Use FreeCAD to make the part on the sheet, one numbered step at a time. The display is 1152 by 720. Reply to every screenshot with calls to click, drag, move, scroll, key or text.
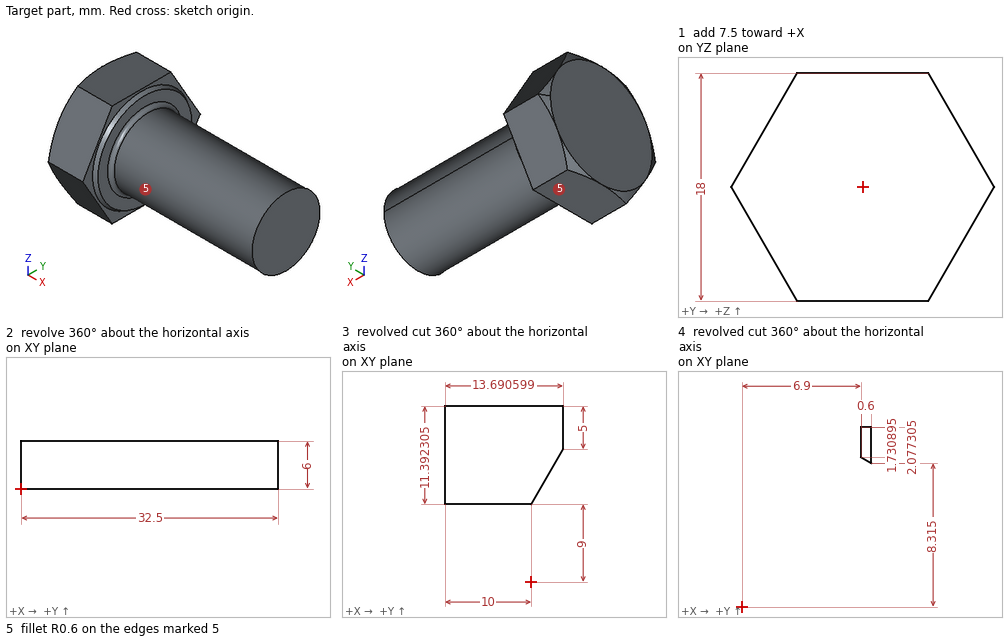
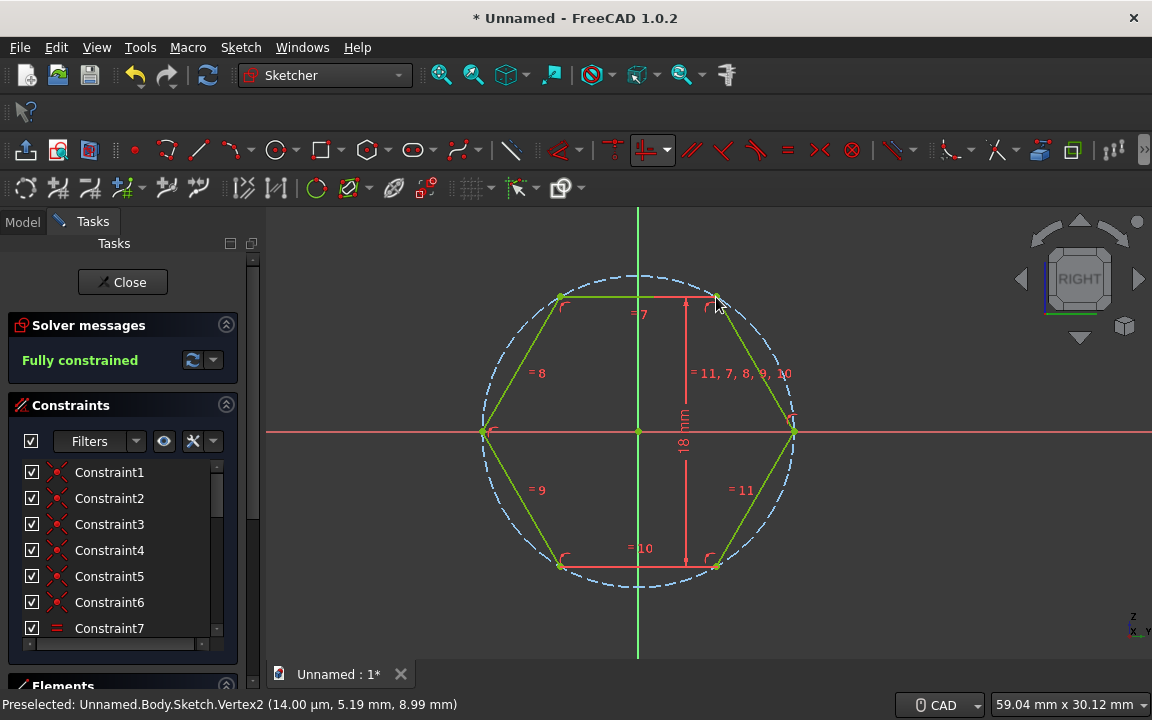
click(123, 282)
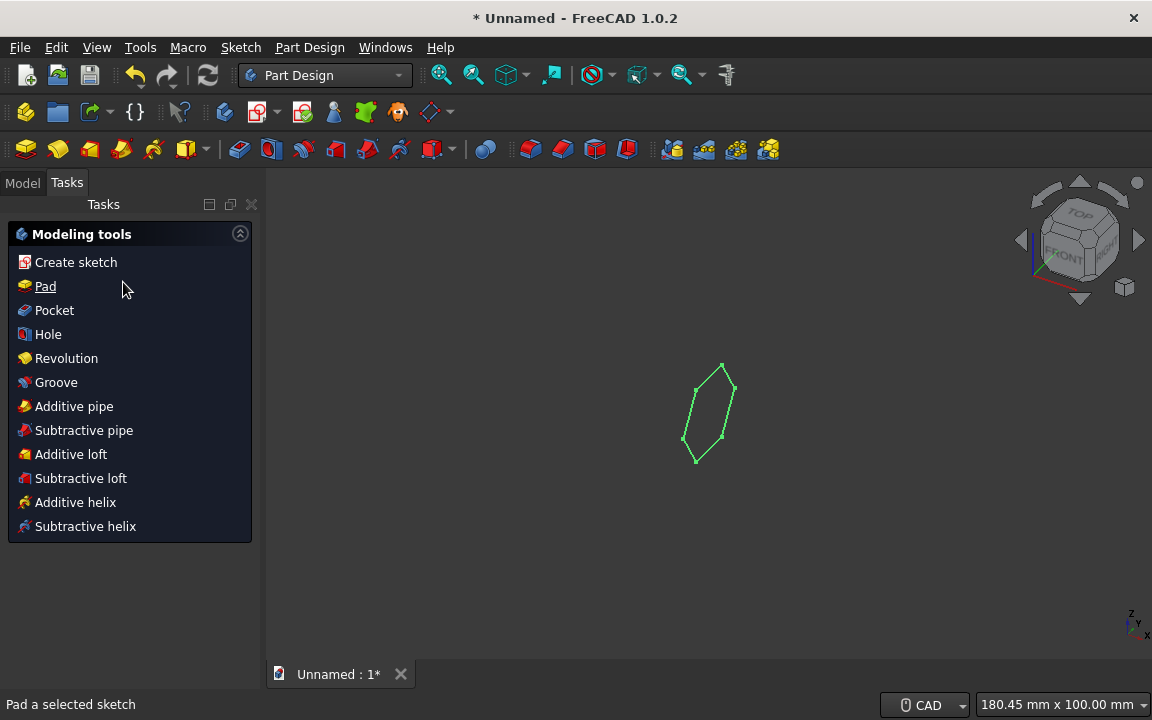
click(26, 150)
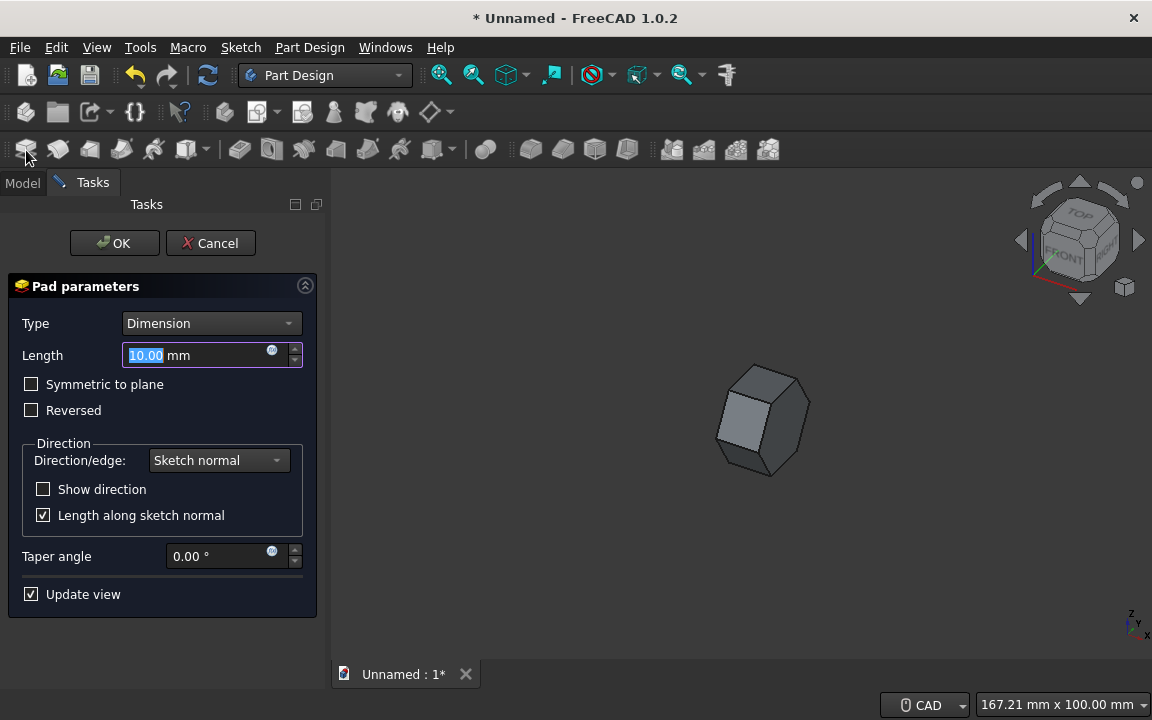
text(7.5)
key(Tab)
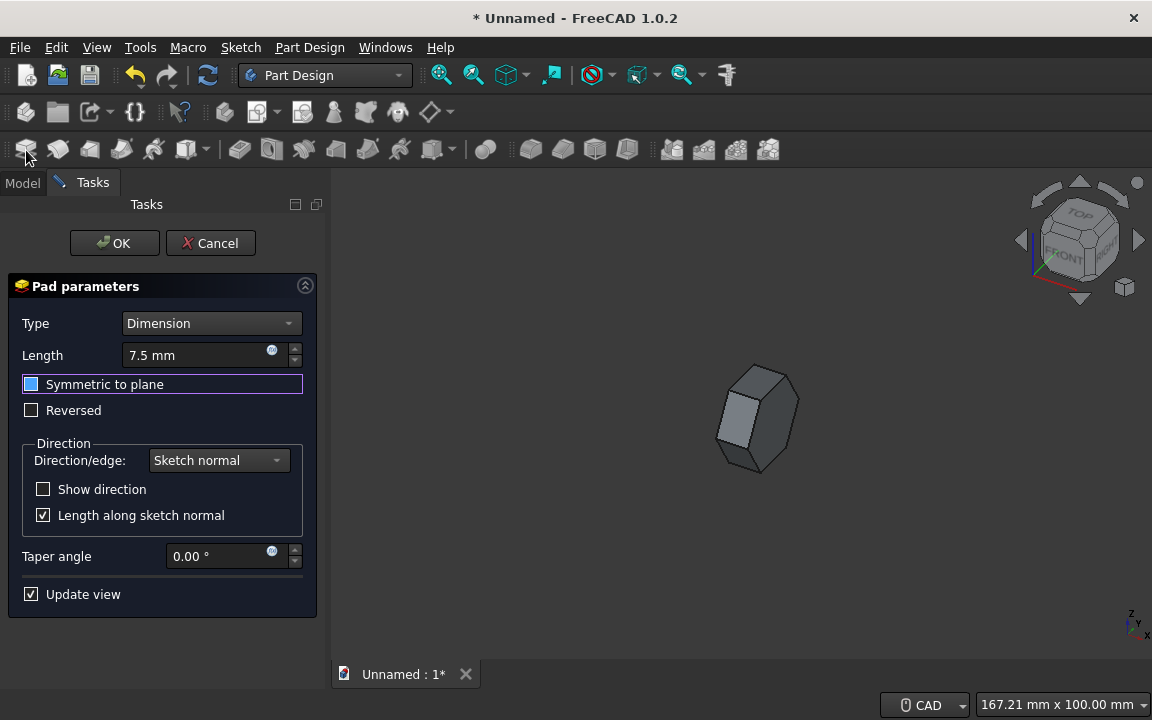
click(115, 243)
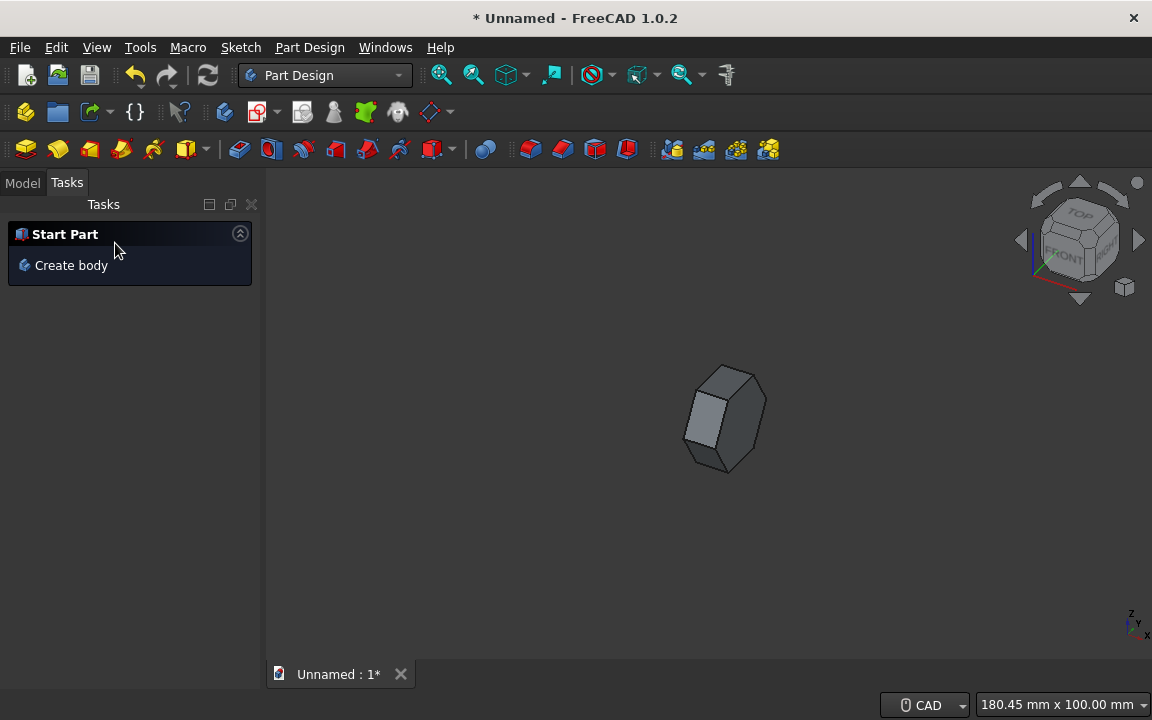
click(442, 76)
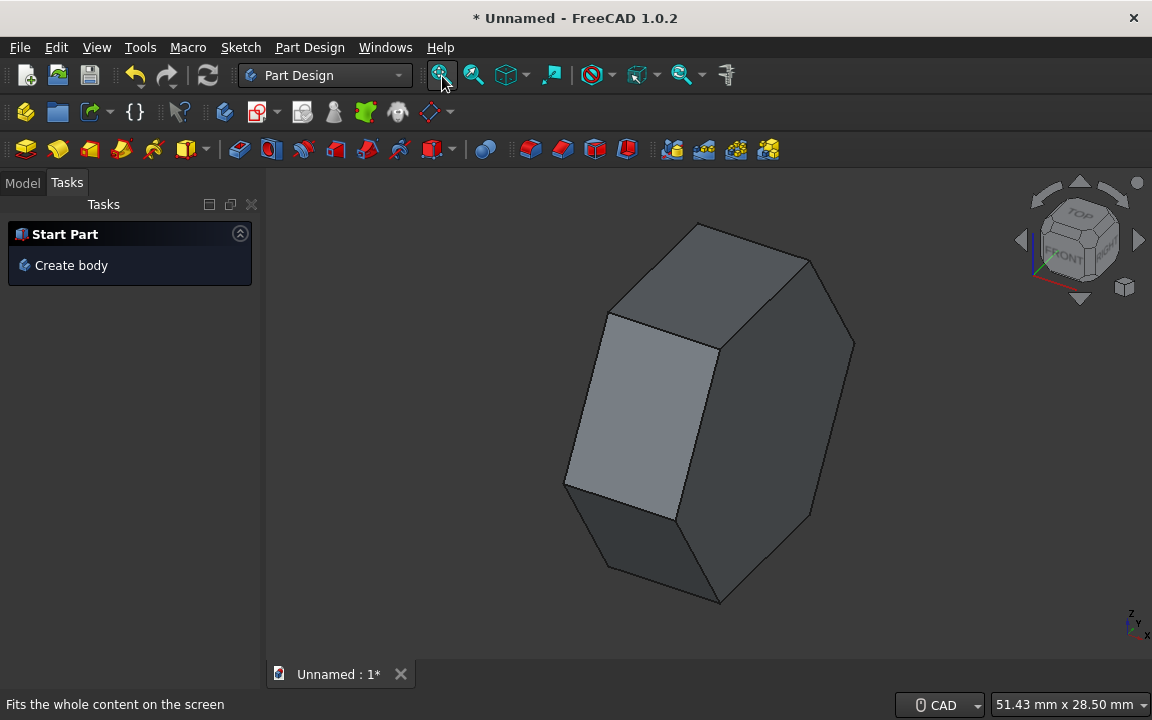
click(258, 112)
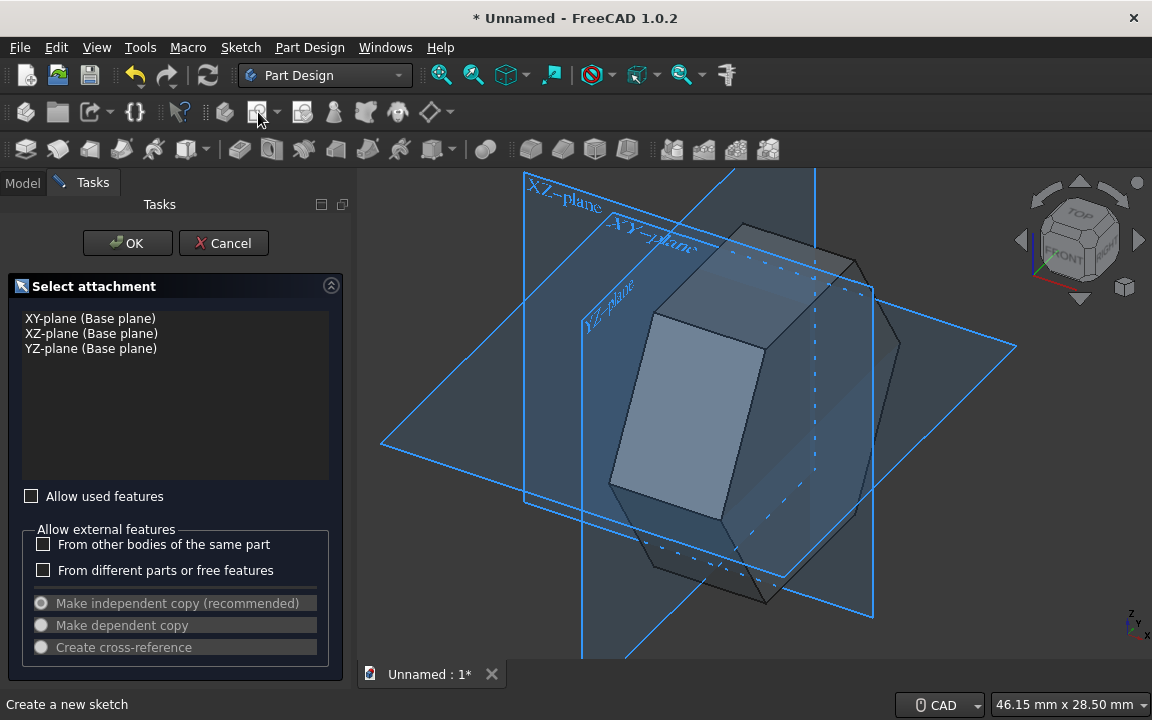
click(82, 318)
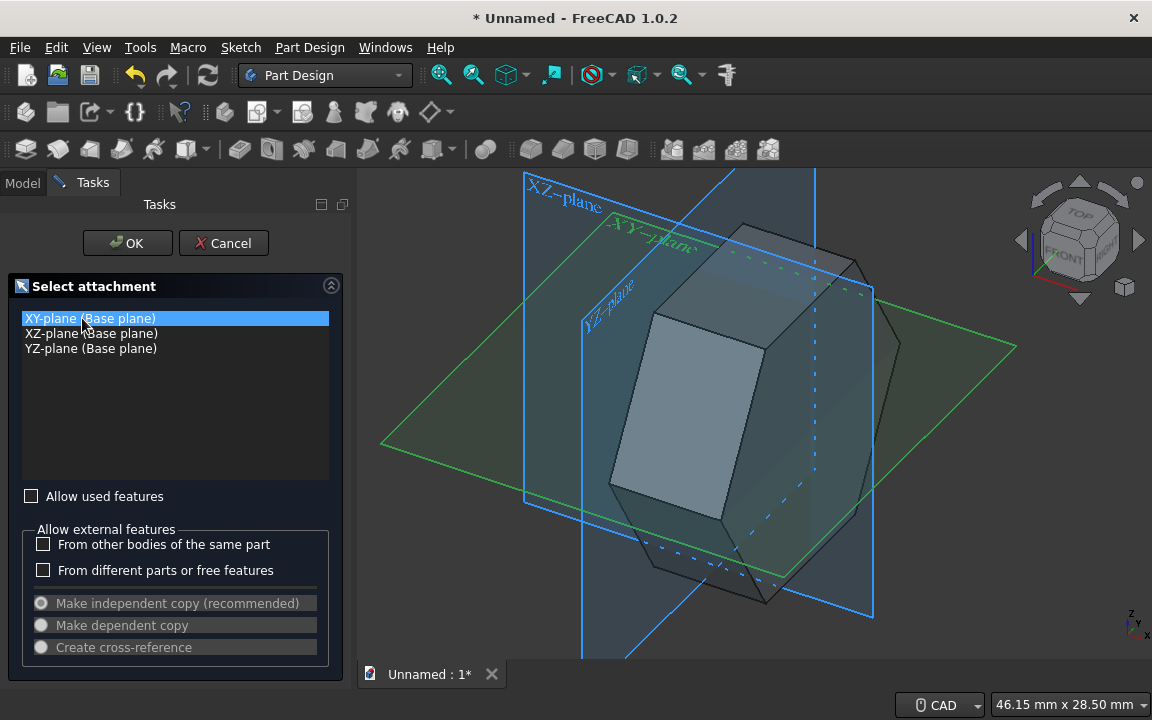
click(128, 243)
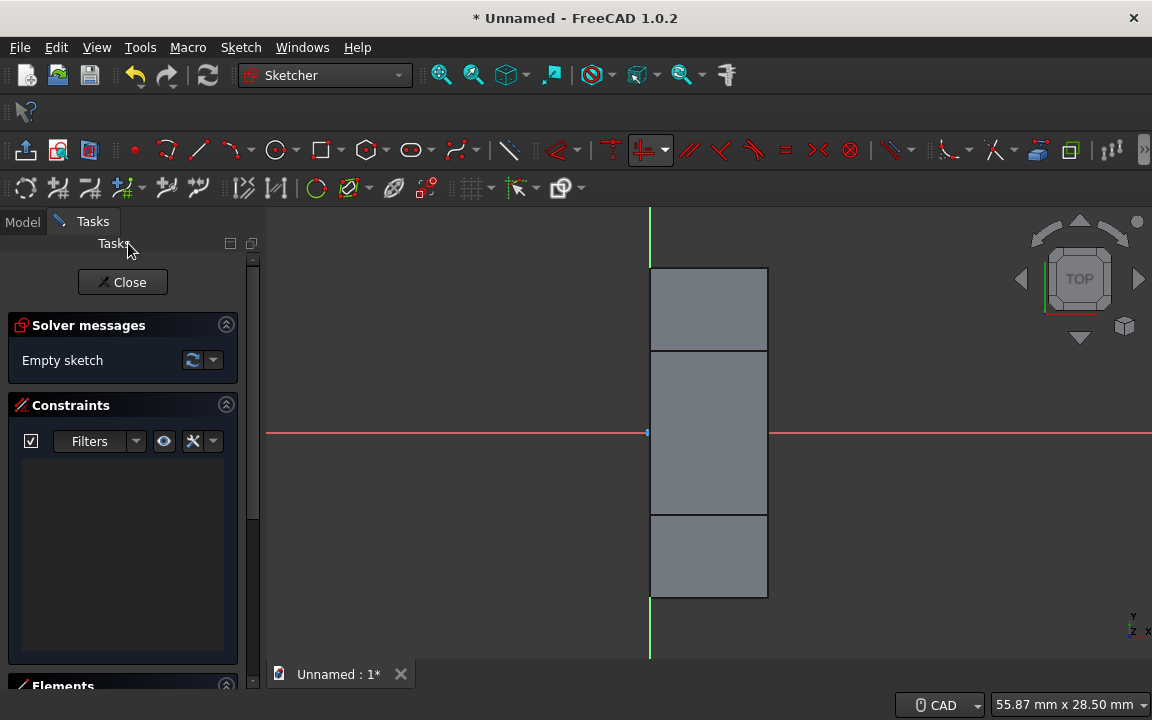
click(90, 150)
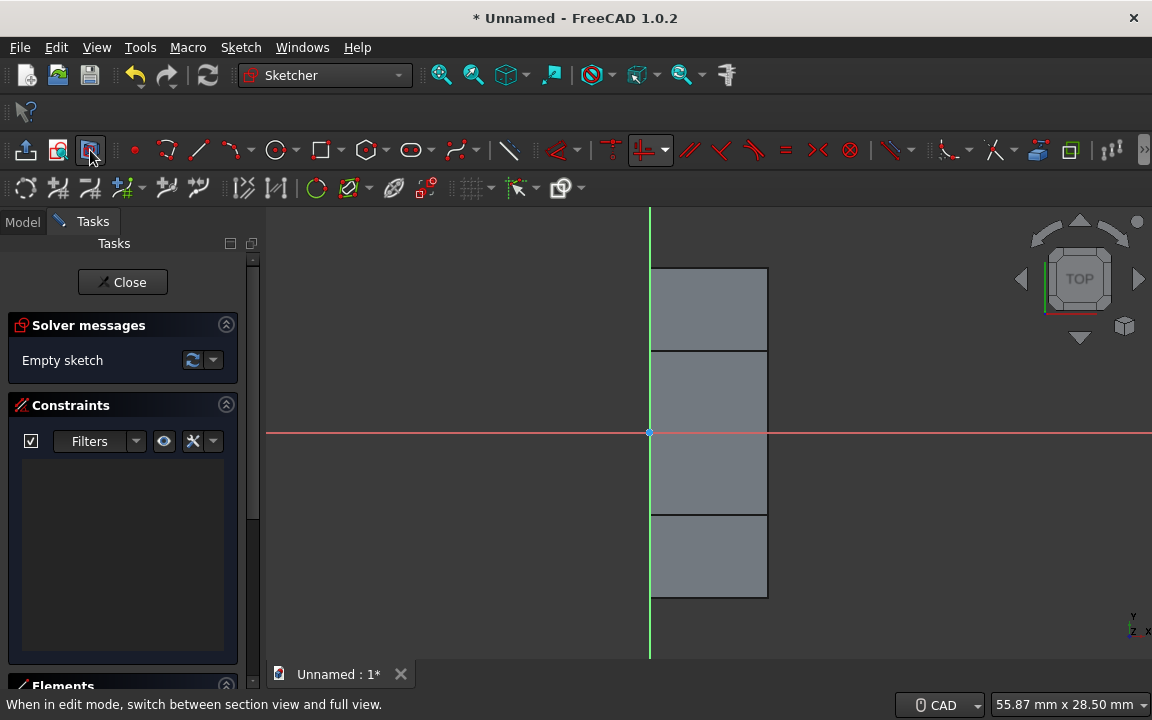
scroll(294, 530, down, 2)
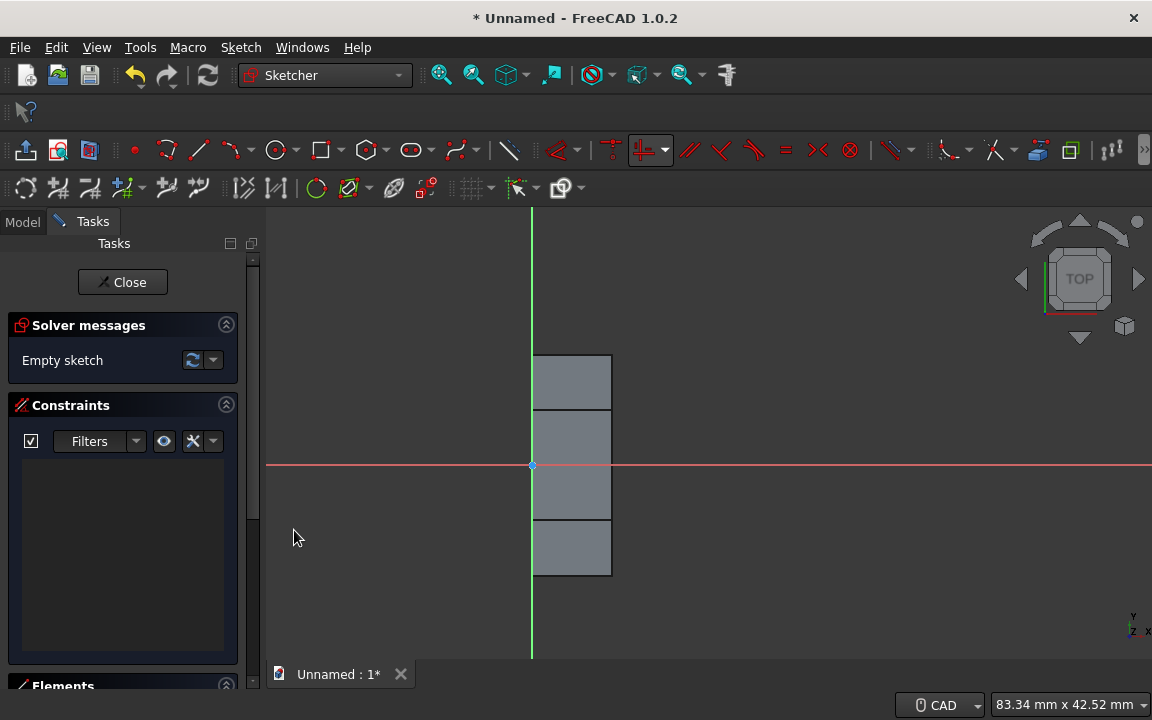
scroll(836, 434, up, 2)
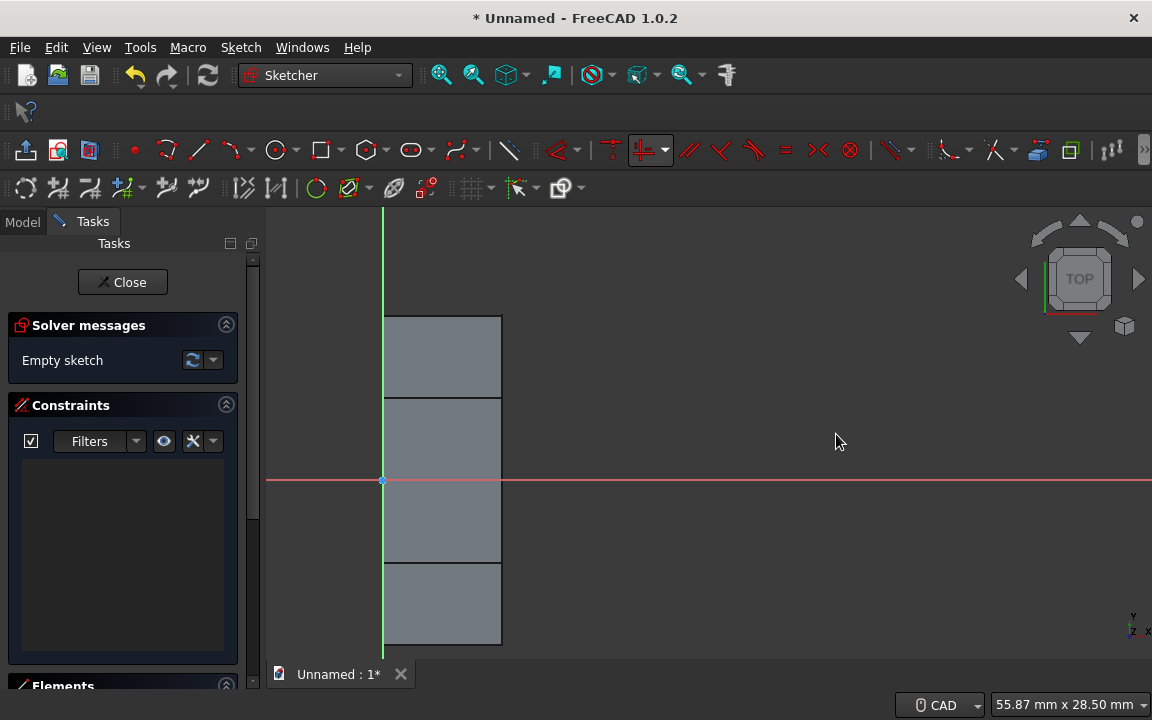
key(g)
key(r)